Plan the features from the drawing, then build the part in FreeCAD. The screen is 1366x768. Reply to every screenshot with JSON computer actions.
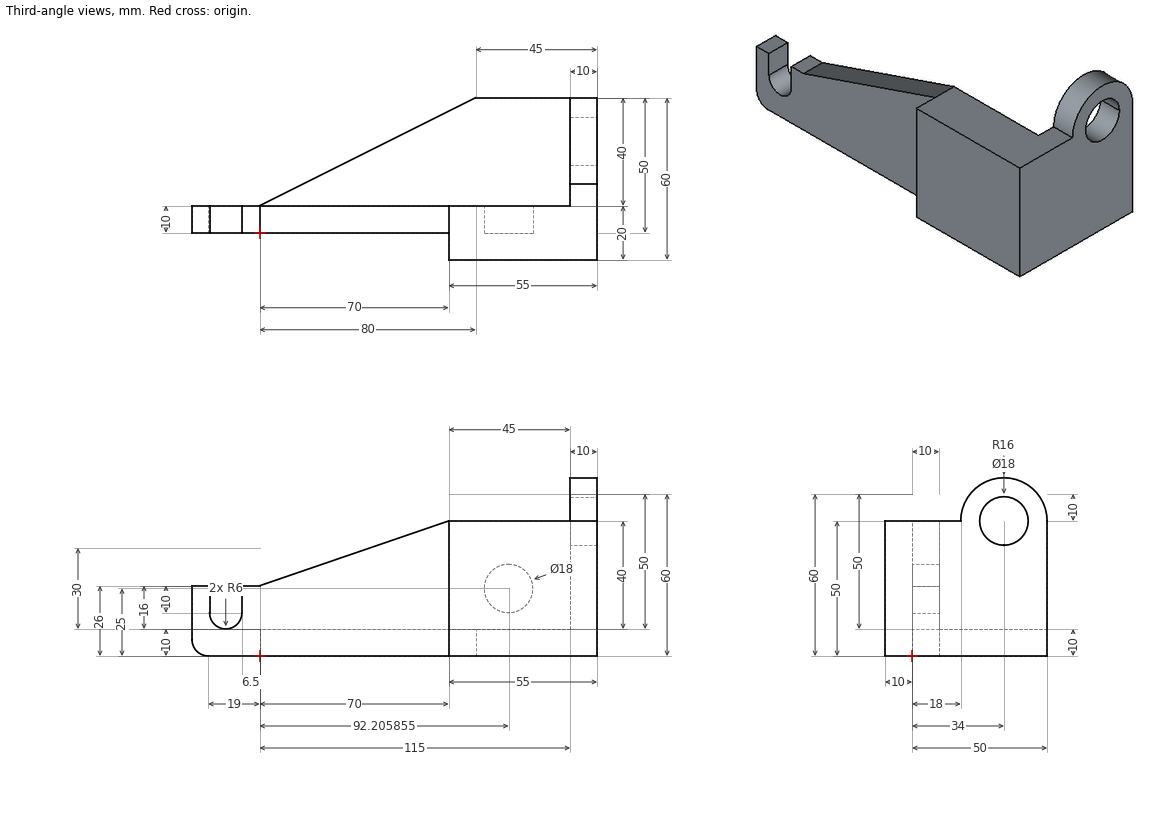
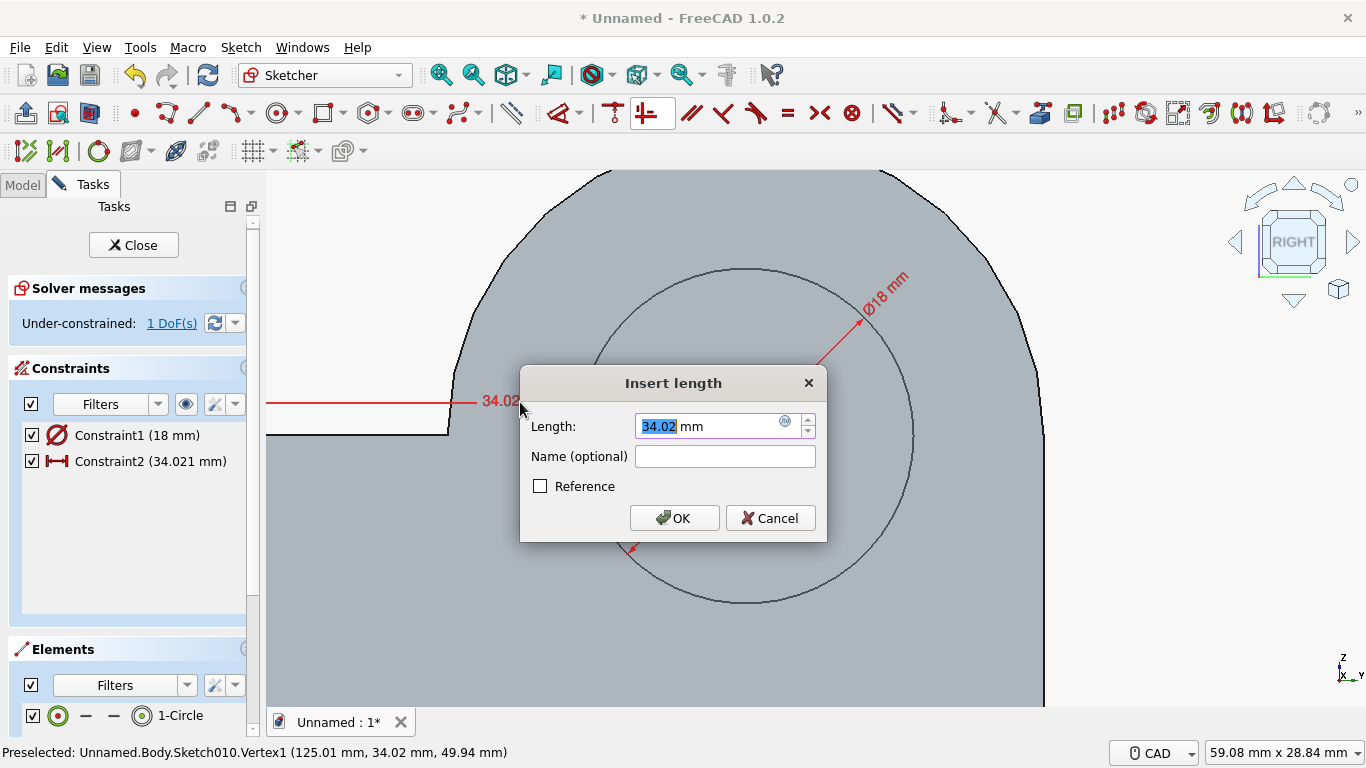
{"action": "type", "text": "34"}
{"action": "key", "text": "Return"}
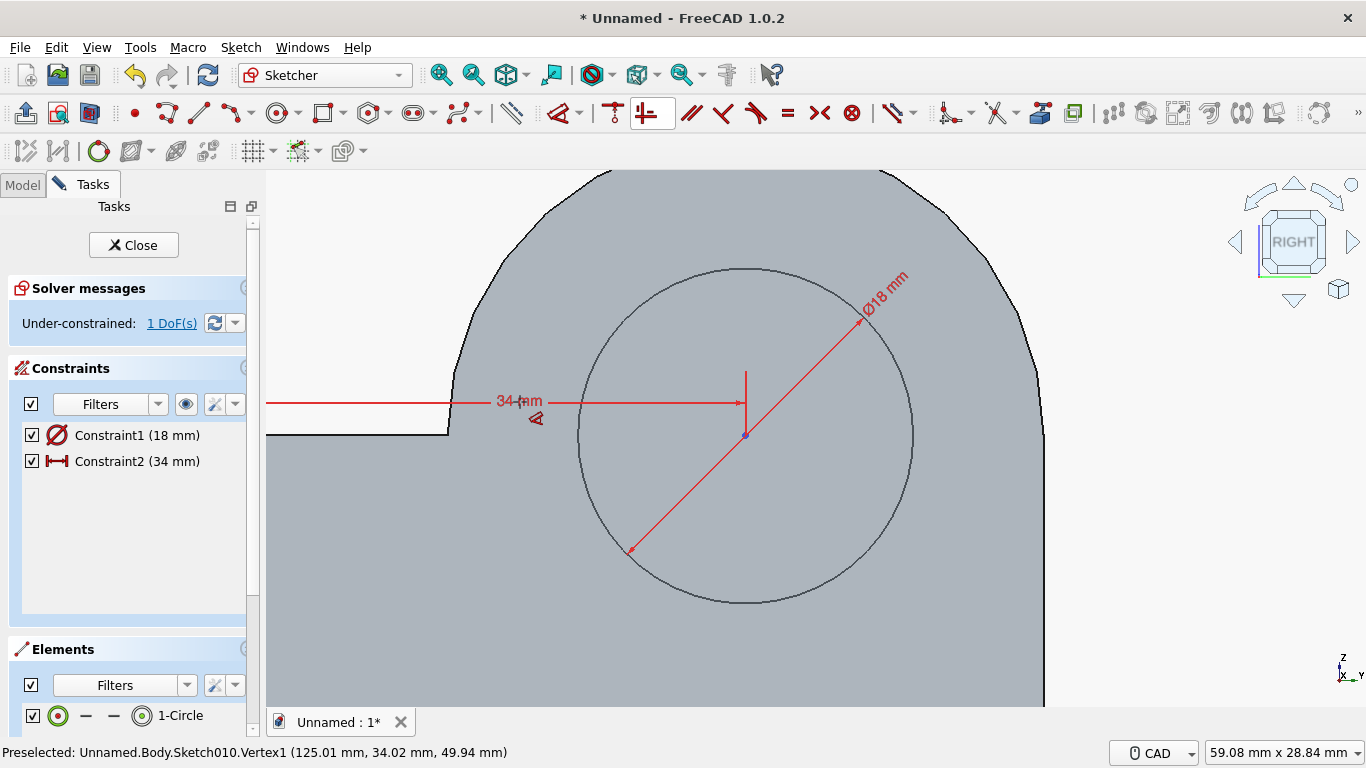
{"action": "left_click", "coordinate": [746, 436]}
{"action": "left_click", "coordinate": [780, 558]}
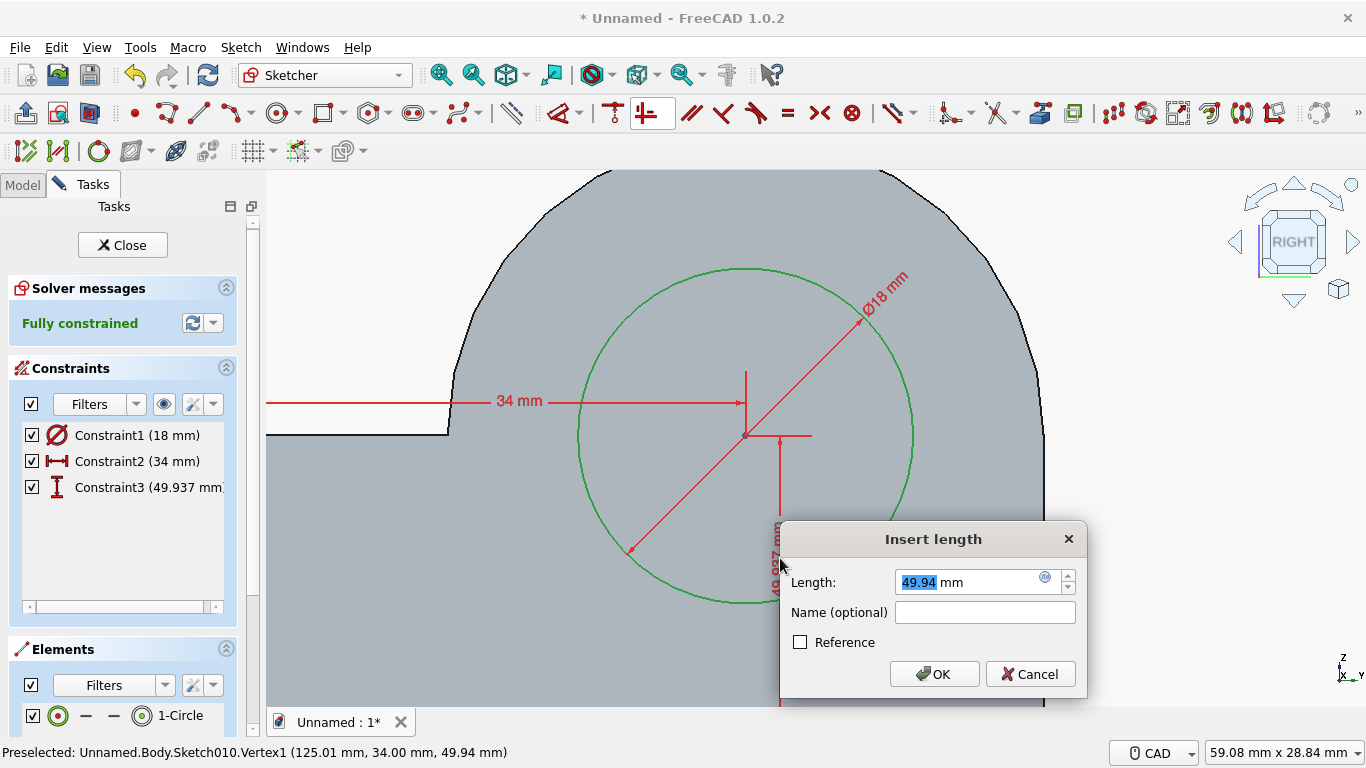
{"action": "type", "text": "50"}
{"action": "key", "text": "Return"}
{"action": "key", "text": "Escape"}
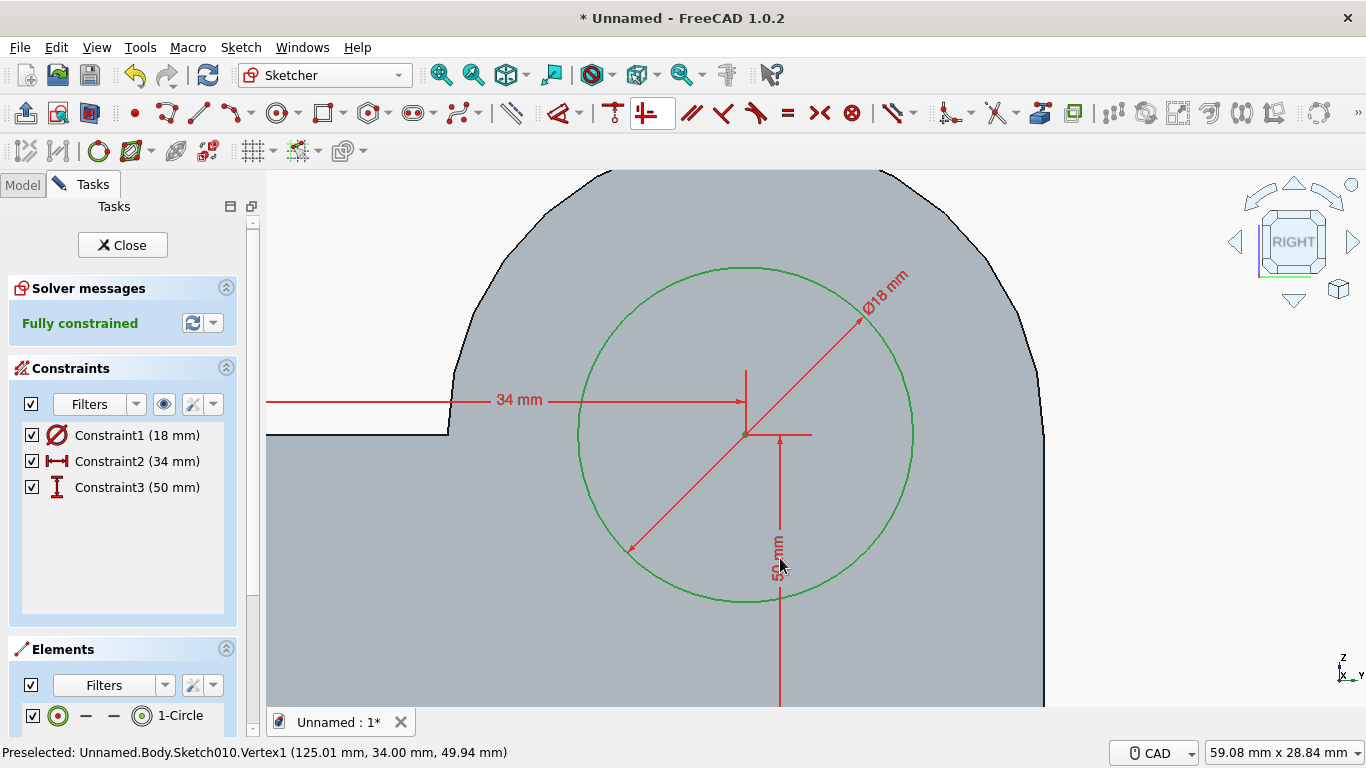
{"action": "left_click", "coordinate": [123, 245]}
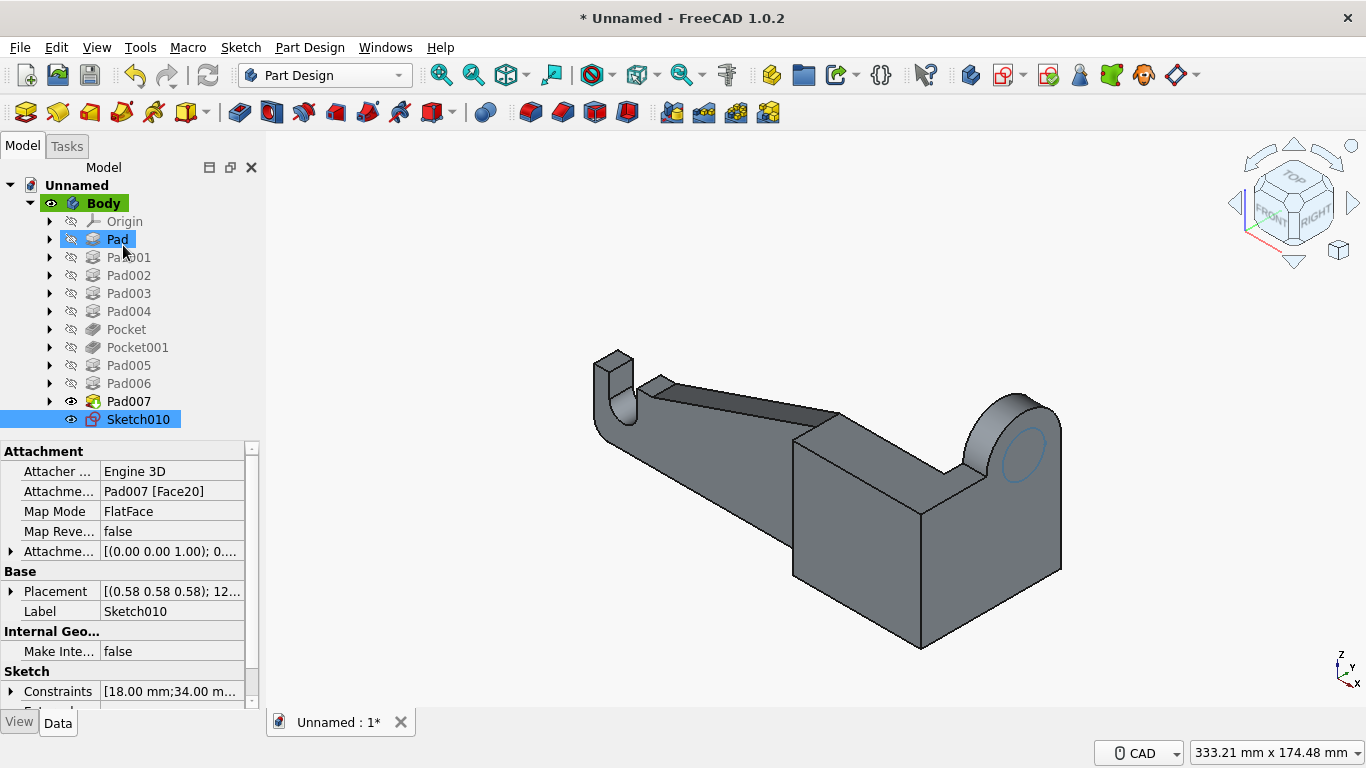
{"action": "left_click", "coordinate": [240, 112]}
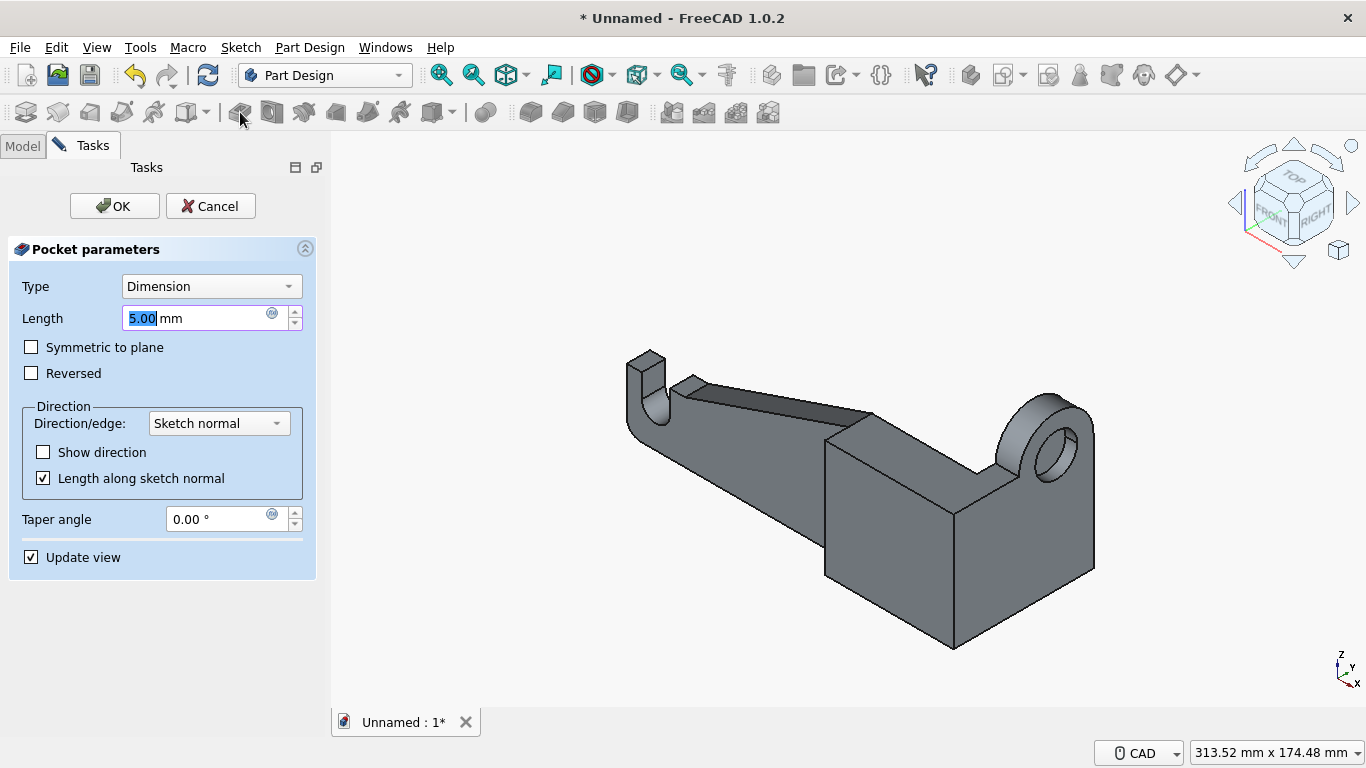
{"action": "type", "text": "10"}
{"action": "key", "text": "Tab"}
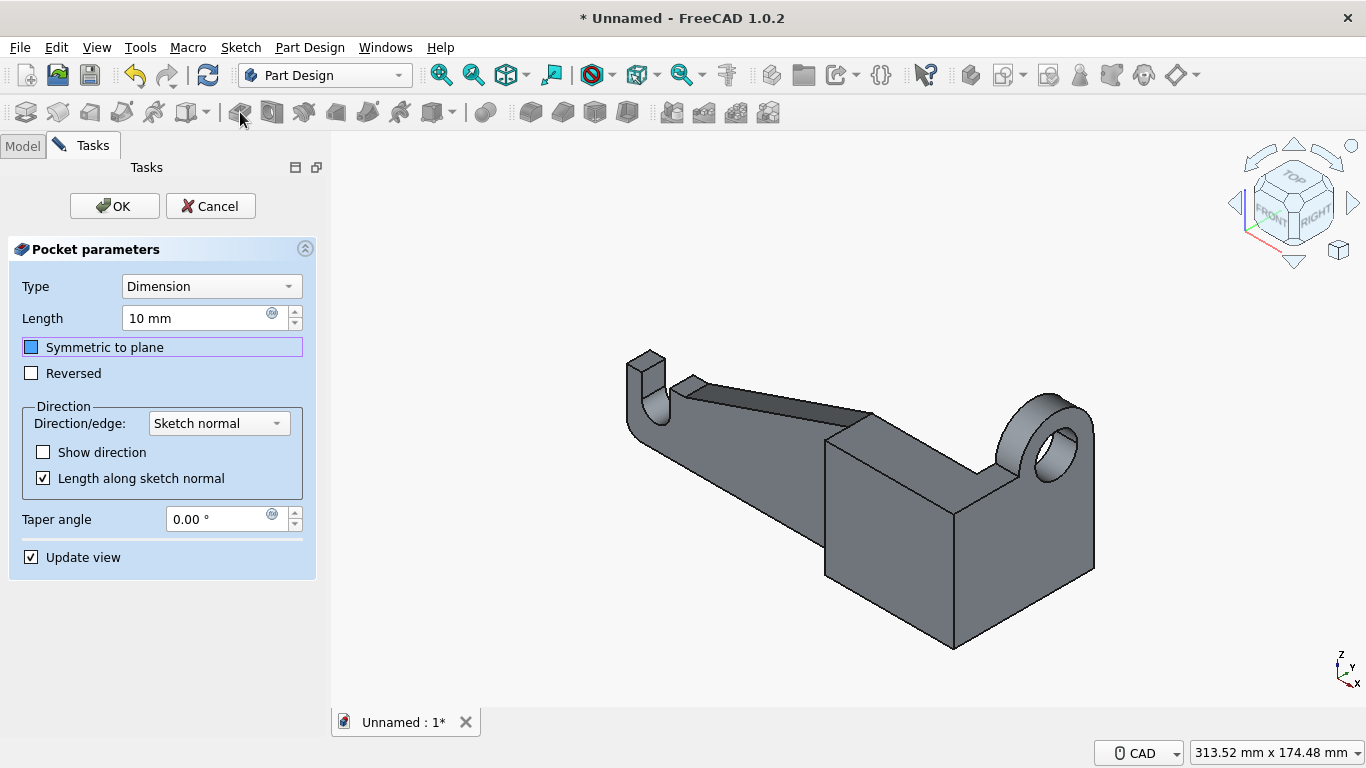
{"action": "left_click", "coordinate": [115, 206]}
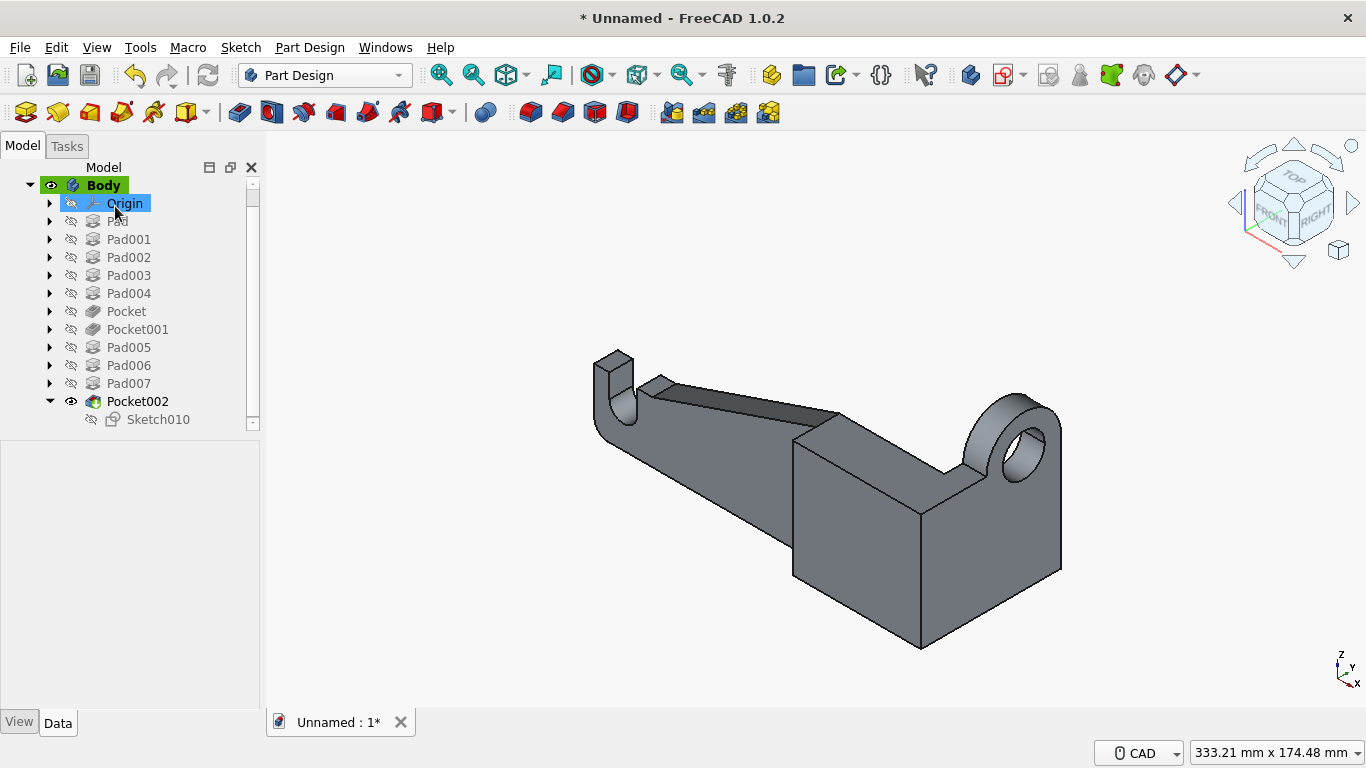
{"action": "key", "text": "4"}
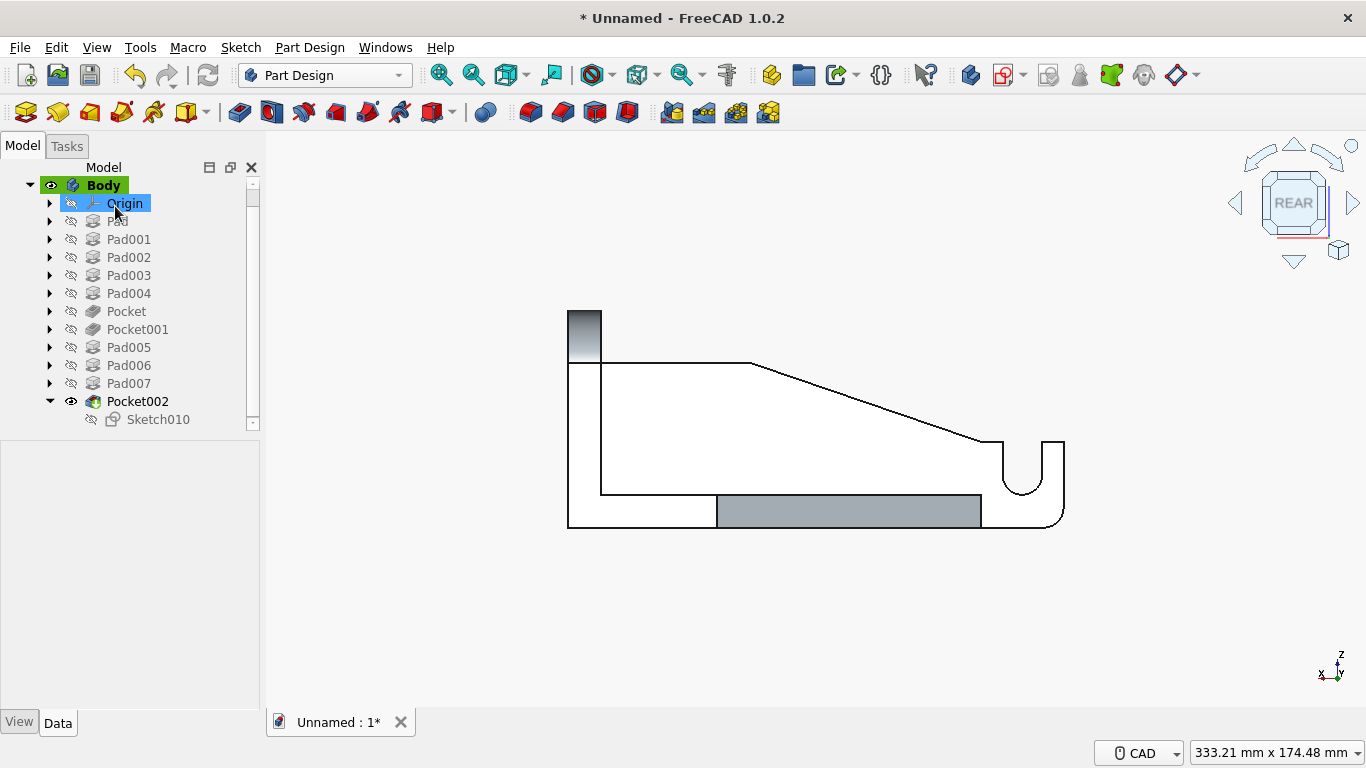
{"action": "left_click", "coordinate": [700, 421]}